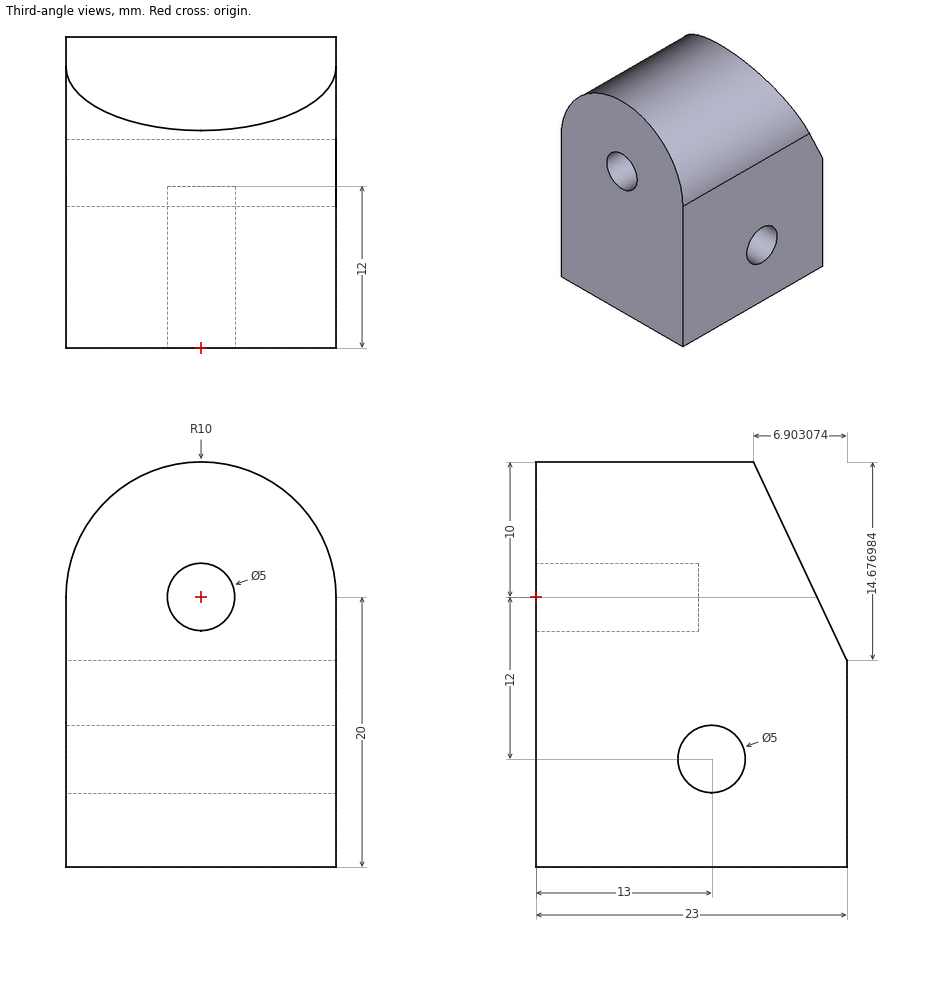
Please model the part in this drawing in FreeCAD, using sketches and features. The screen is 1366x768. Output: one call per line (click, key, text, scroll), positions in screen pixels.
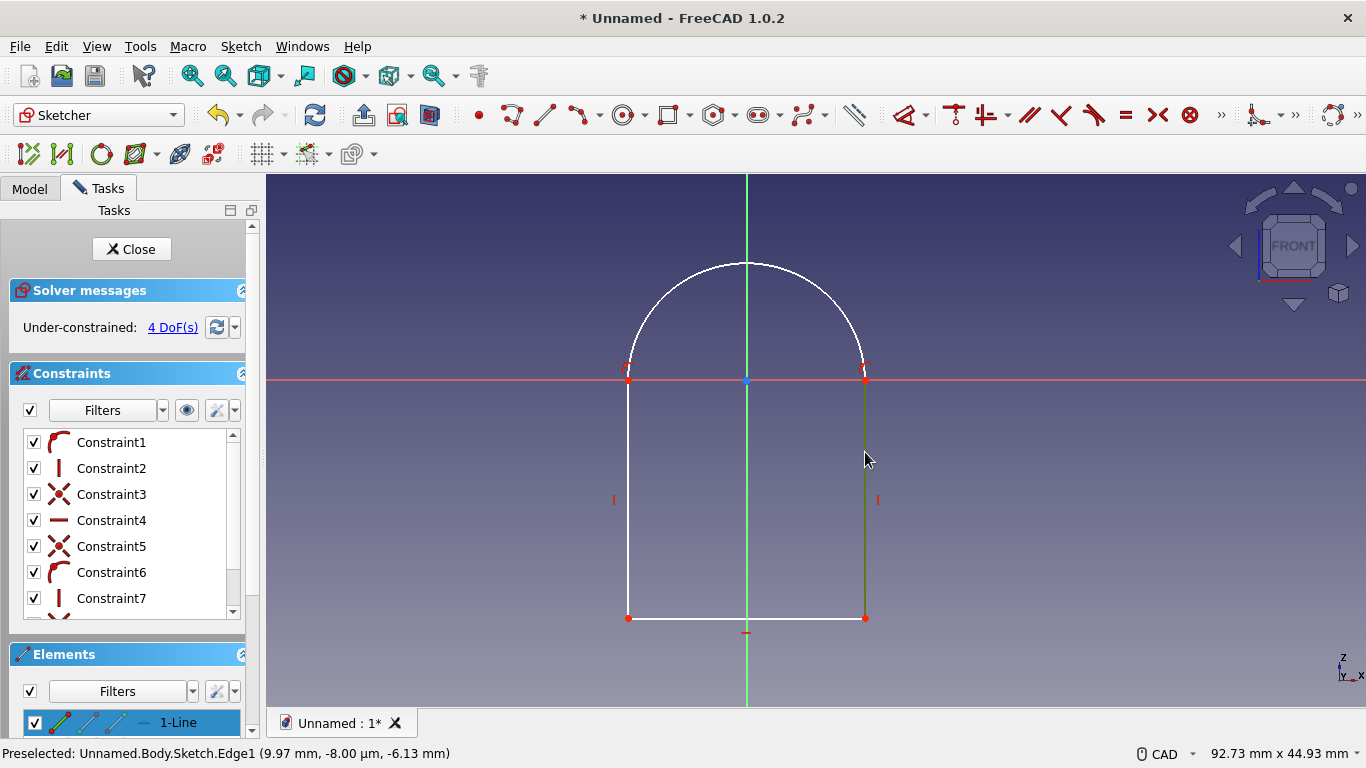
click(816, 286)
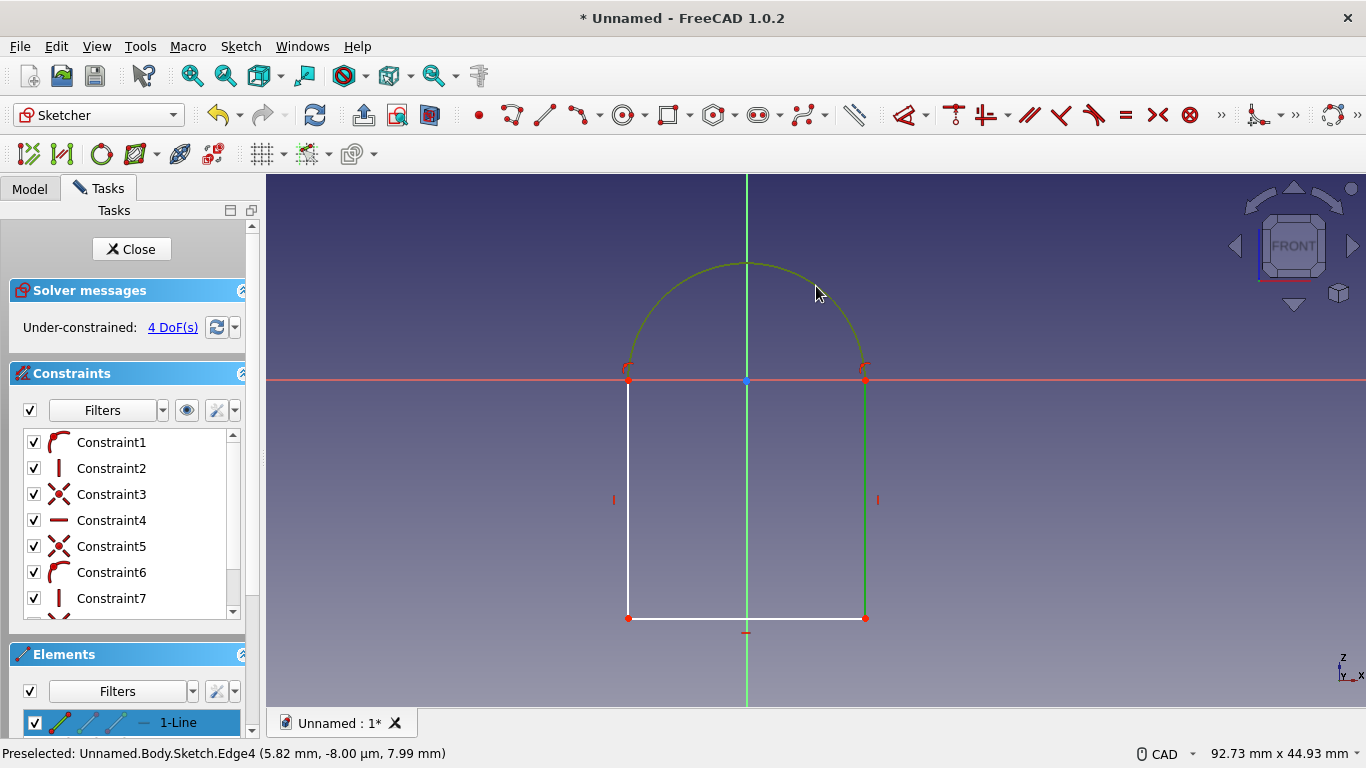
click(1094, 116)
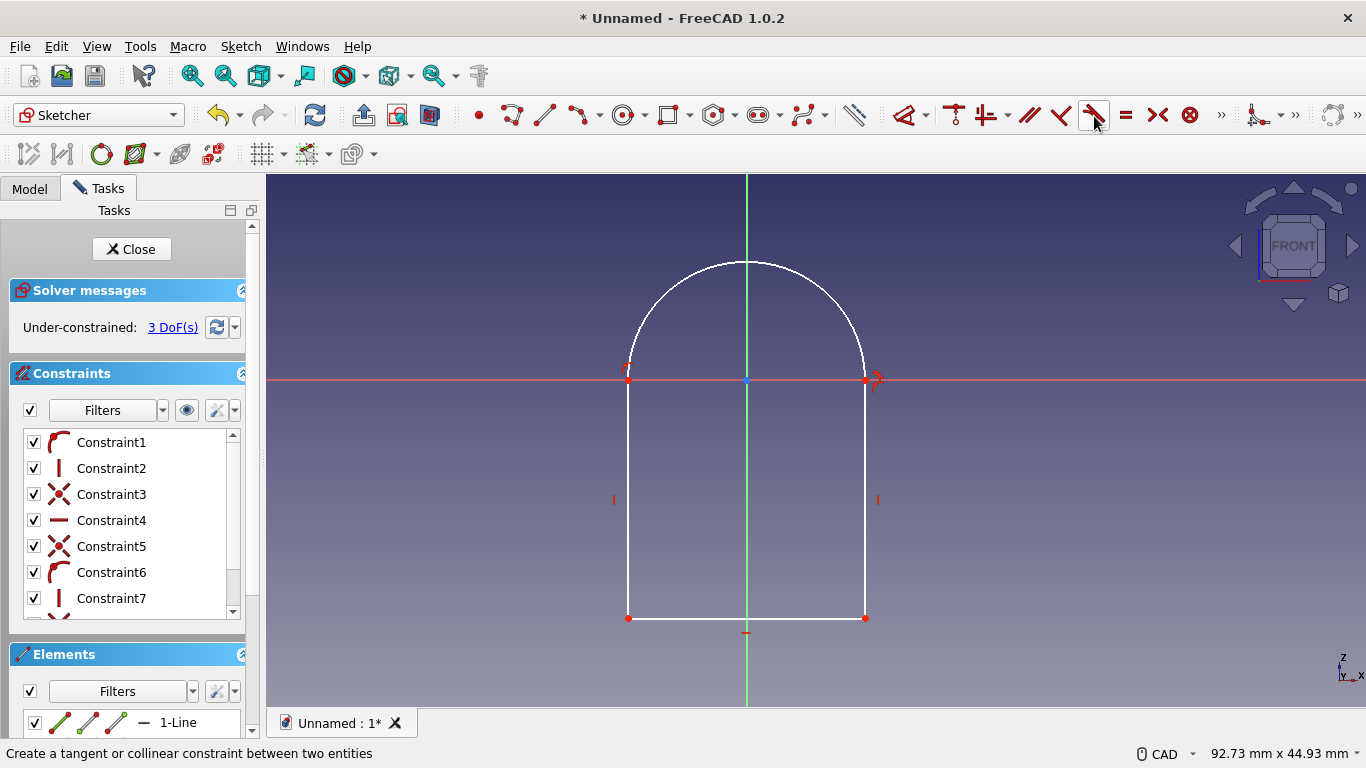
click(747, 380)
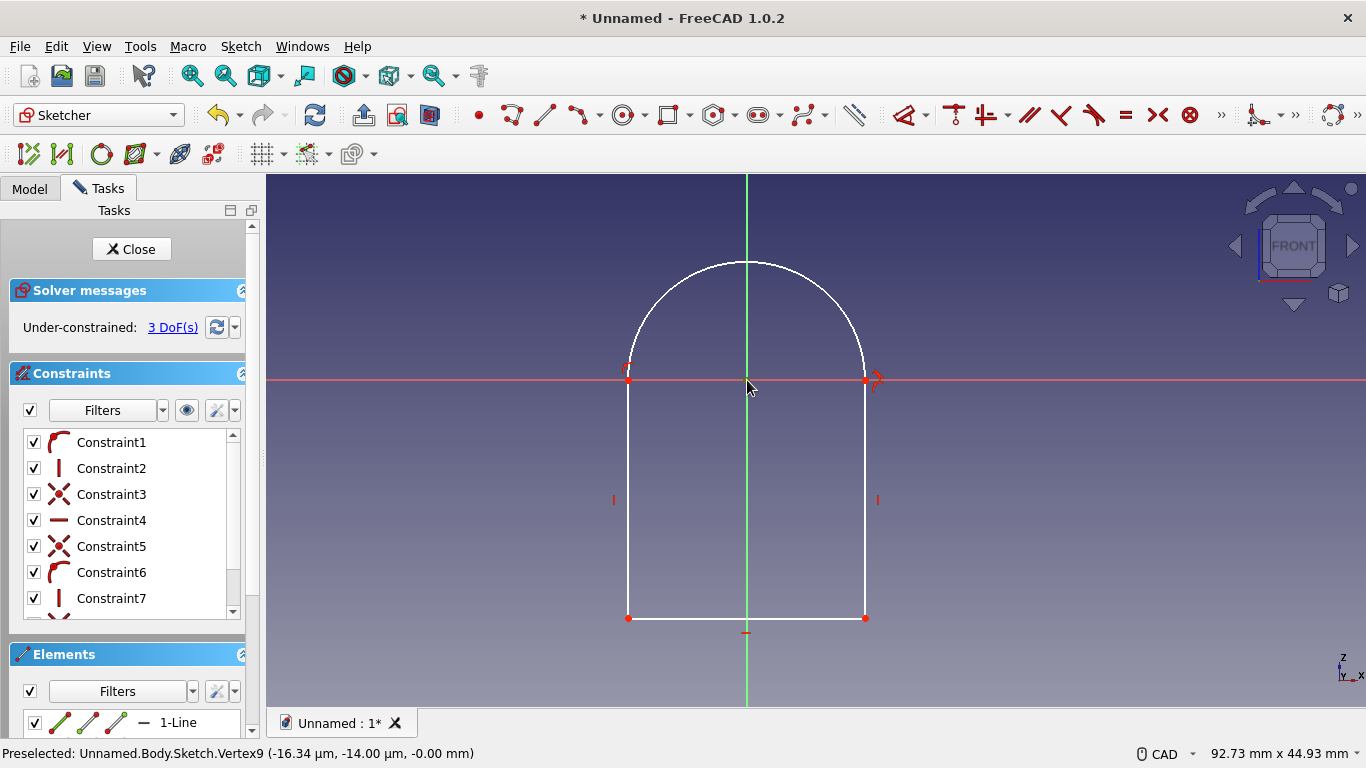
click(747, 577)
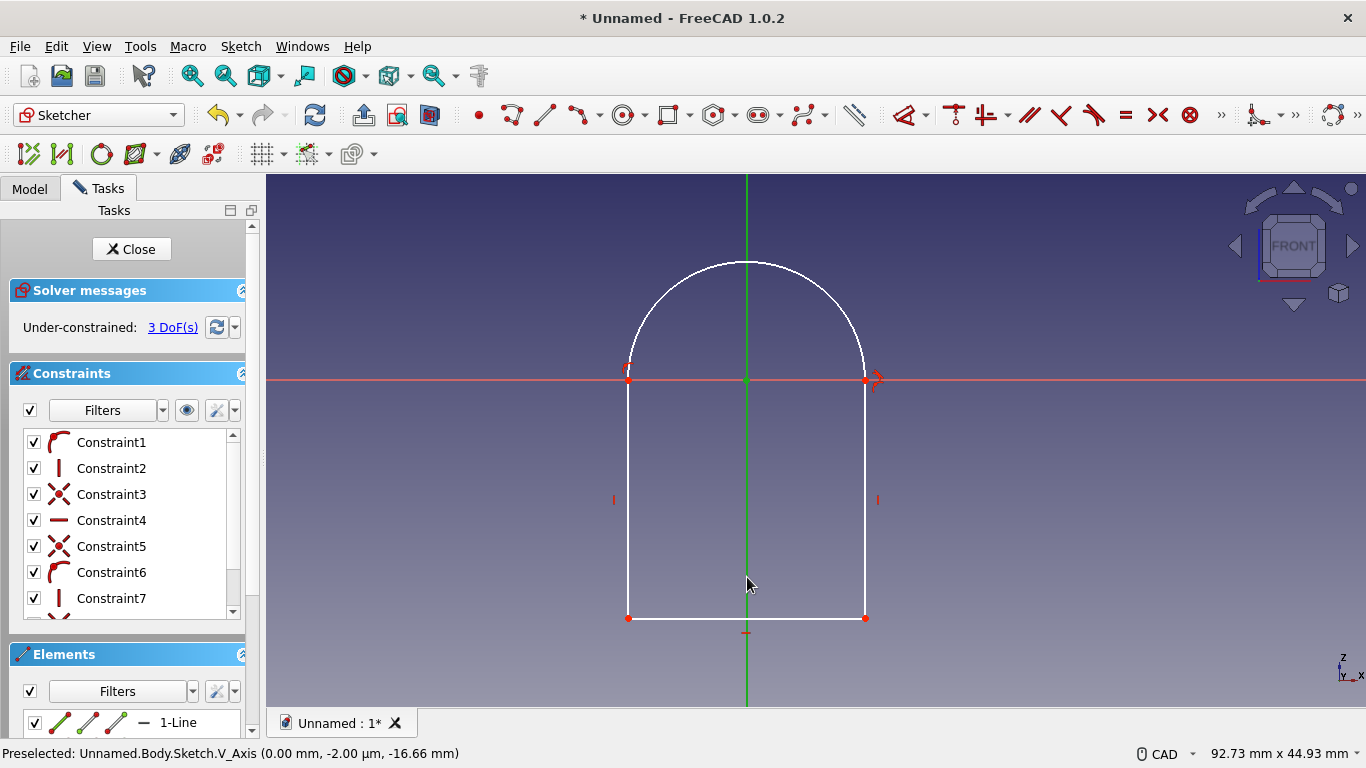
click(954, 116)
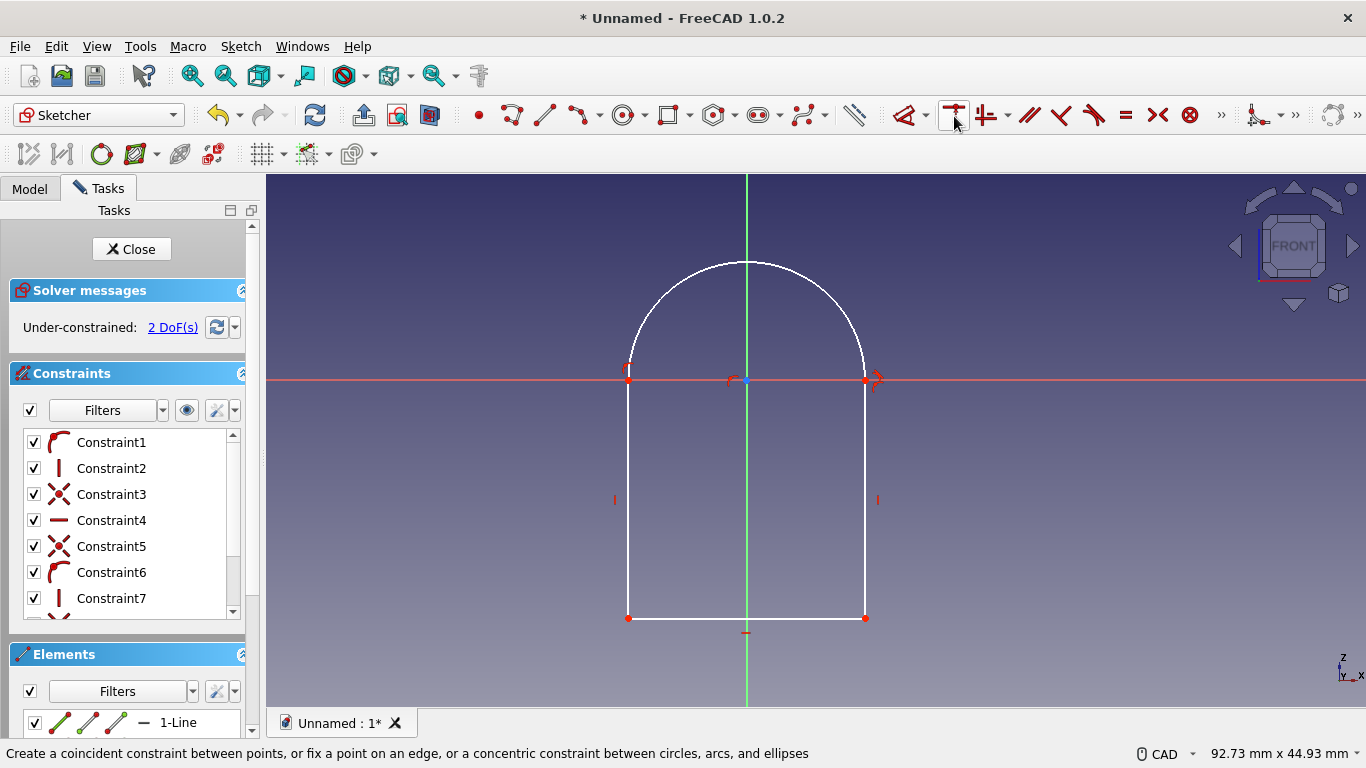
key(d)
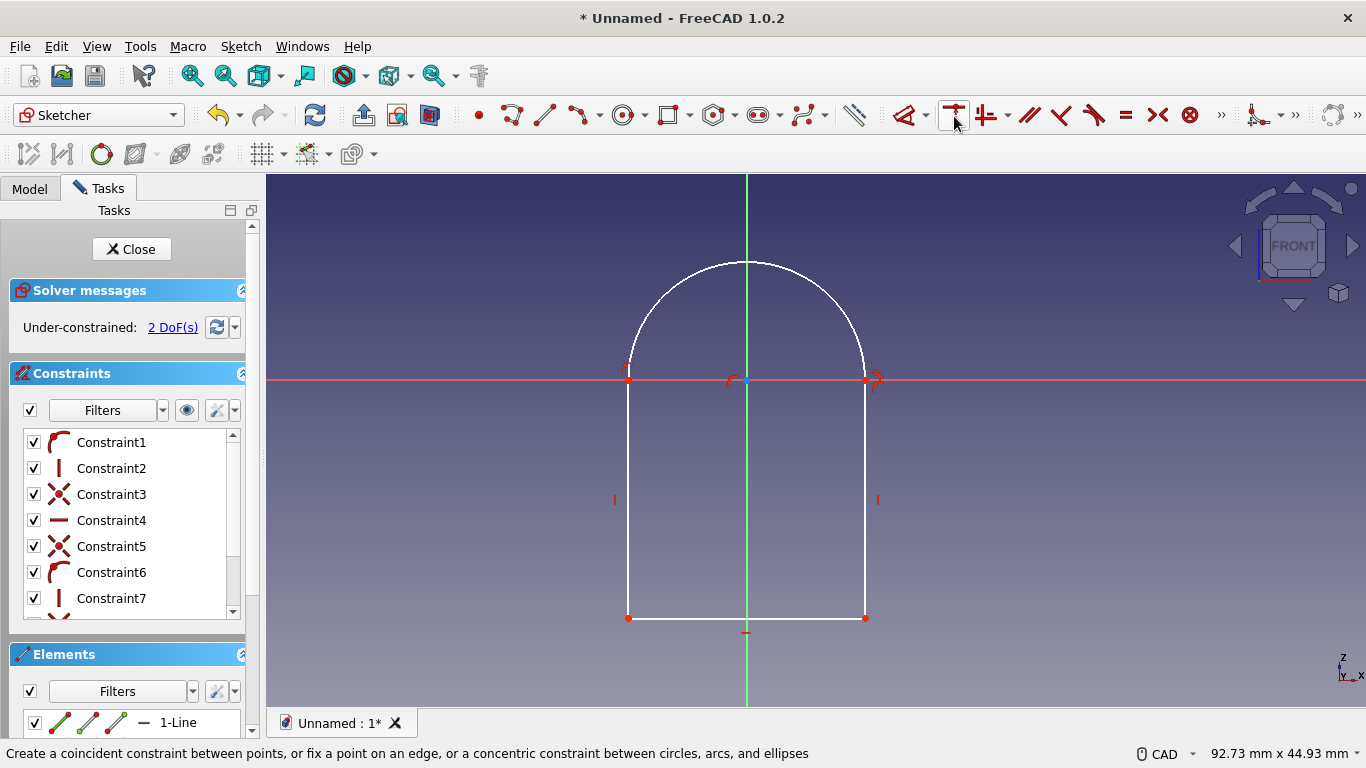
click(816, 285)
click(835, 259)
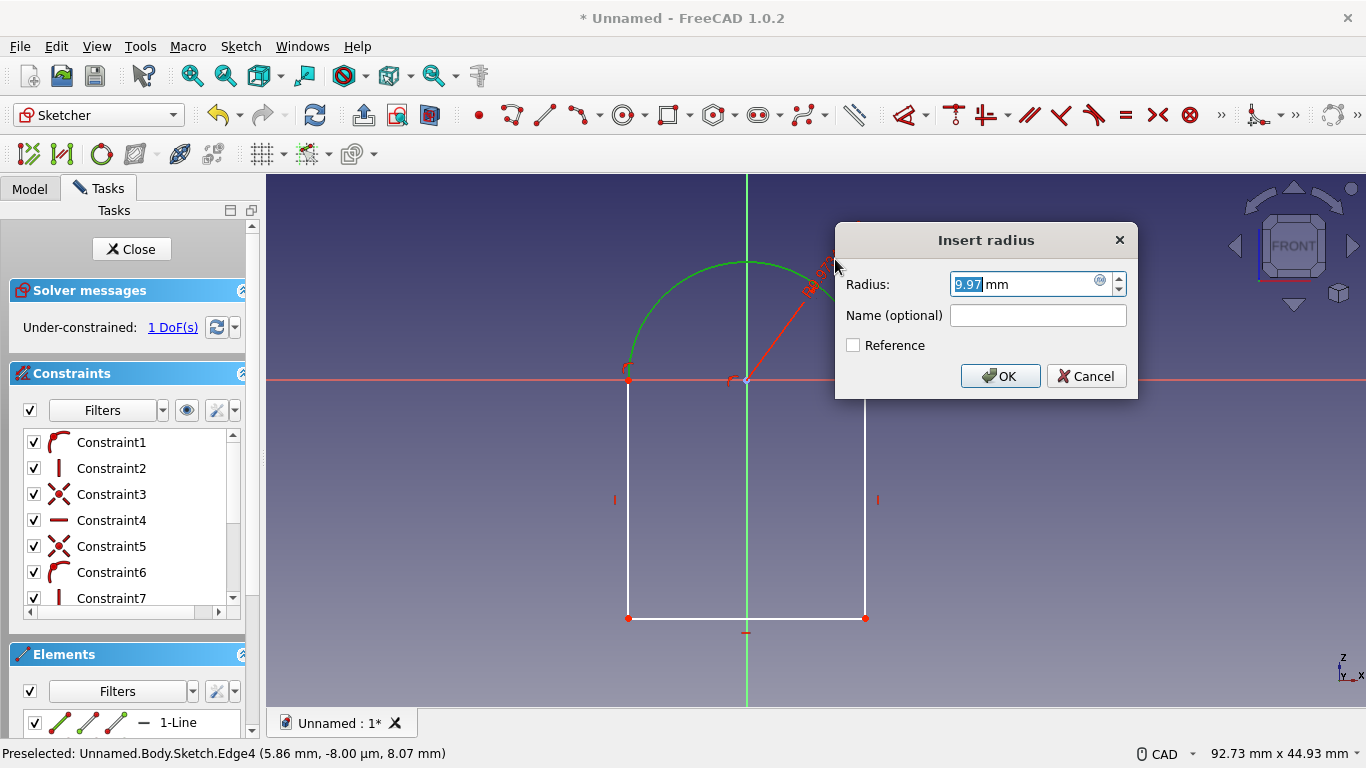
text(10)
key(Return)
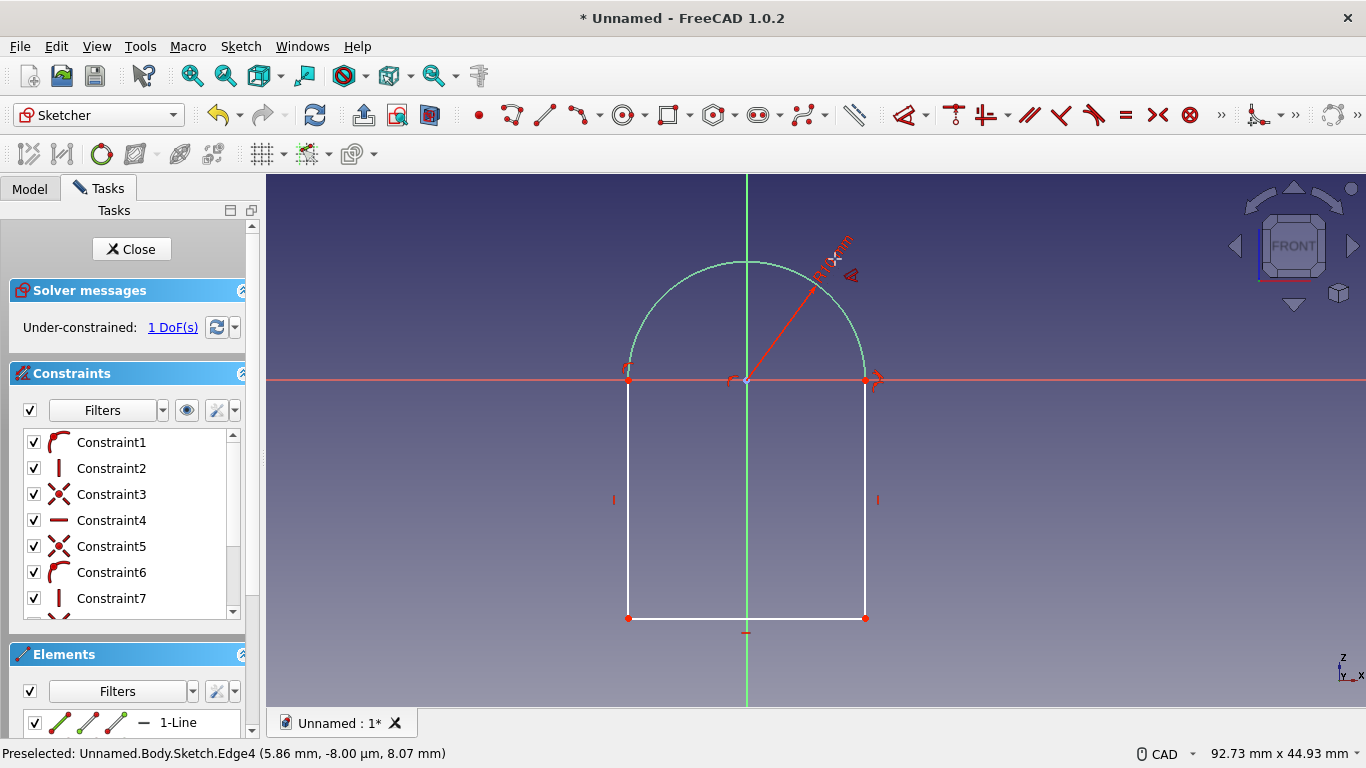
click(865, 452)
click(899, 500)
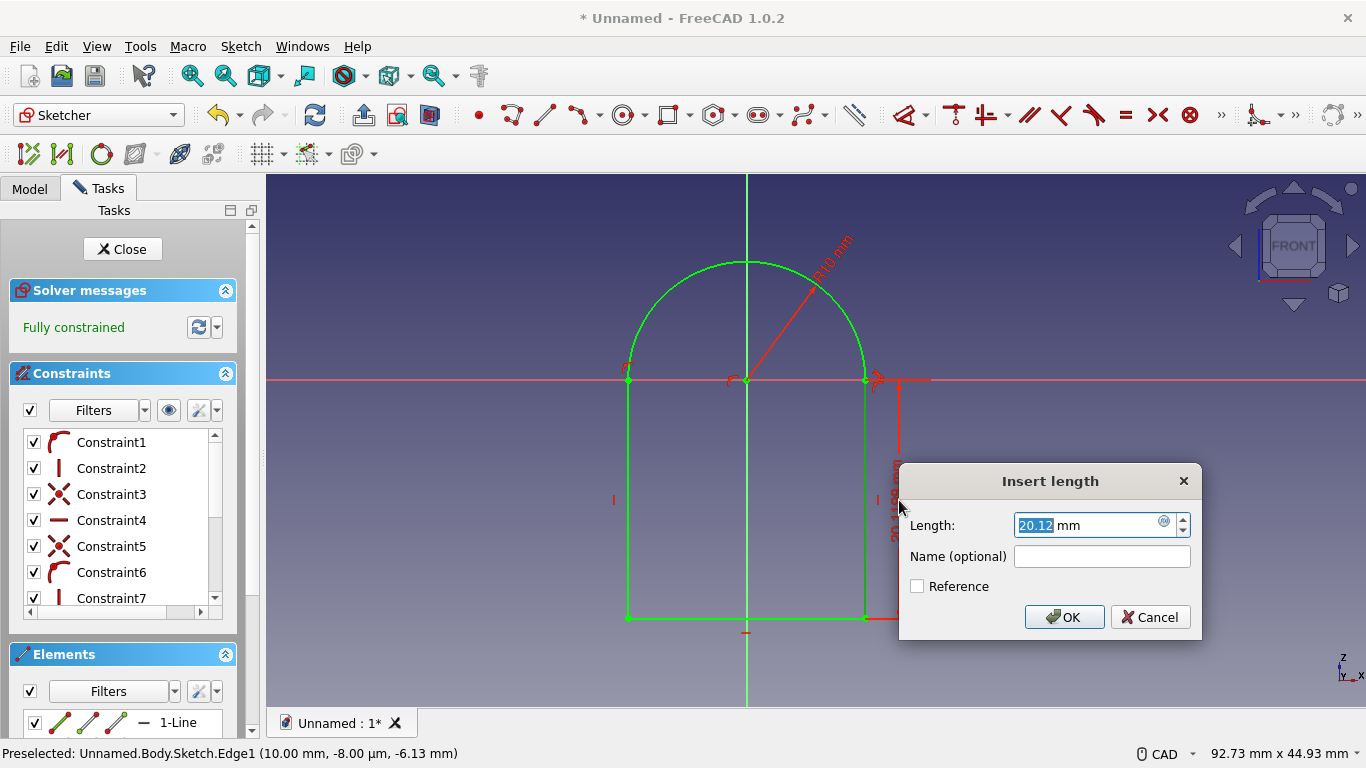
text(20)
key(Return)
key(Escape)